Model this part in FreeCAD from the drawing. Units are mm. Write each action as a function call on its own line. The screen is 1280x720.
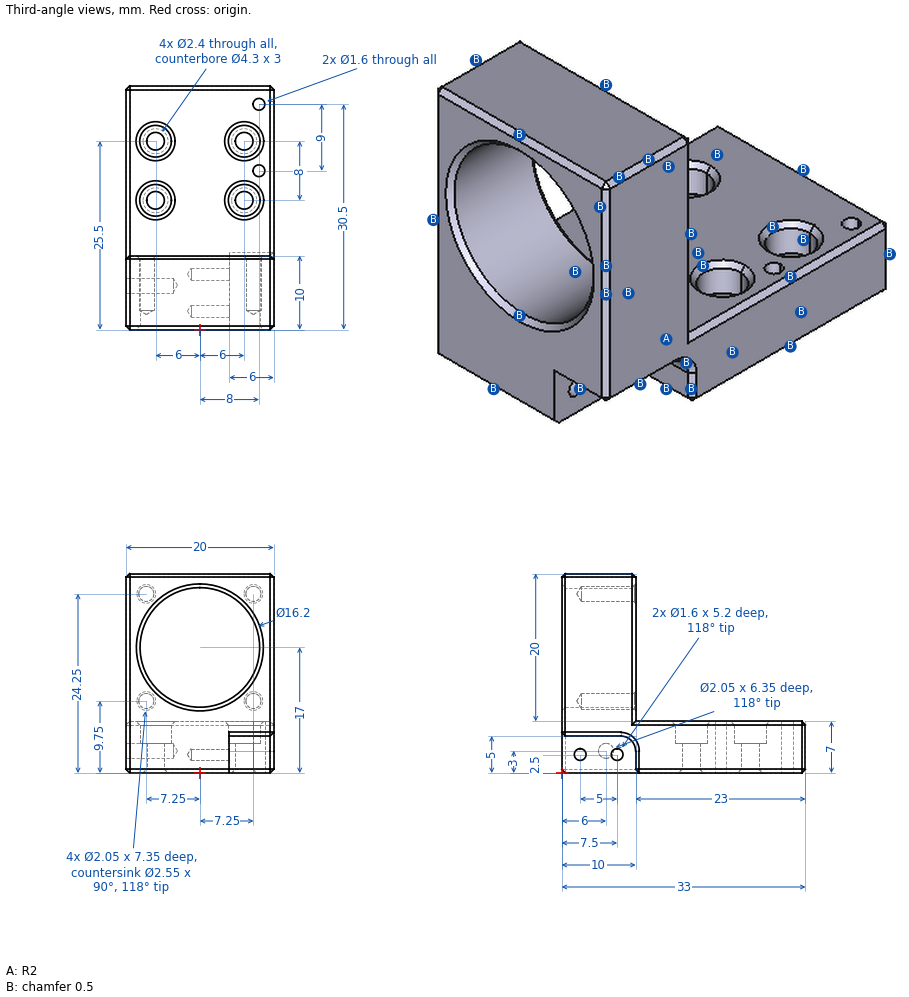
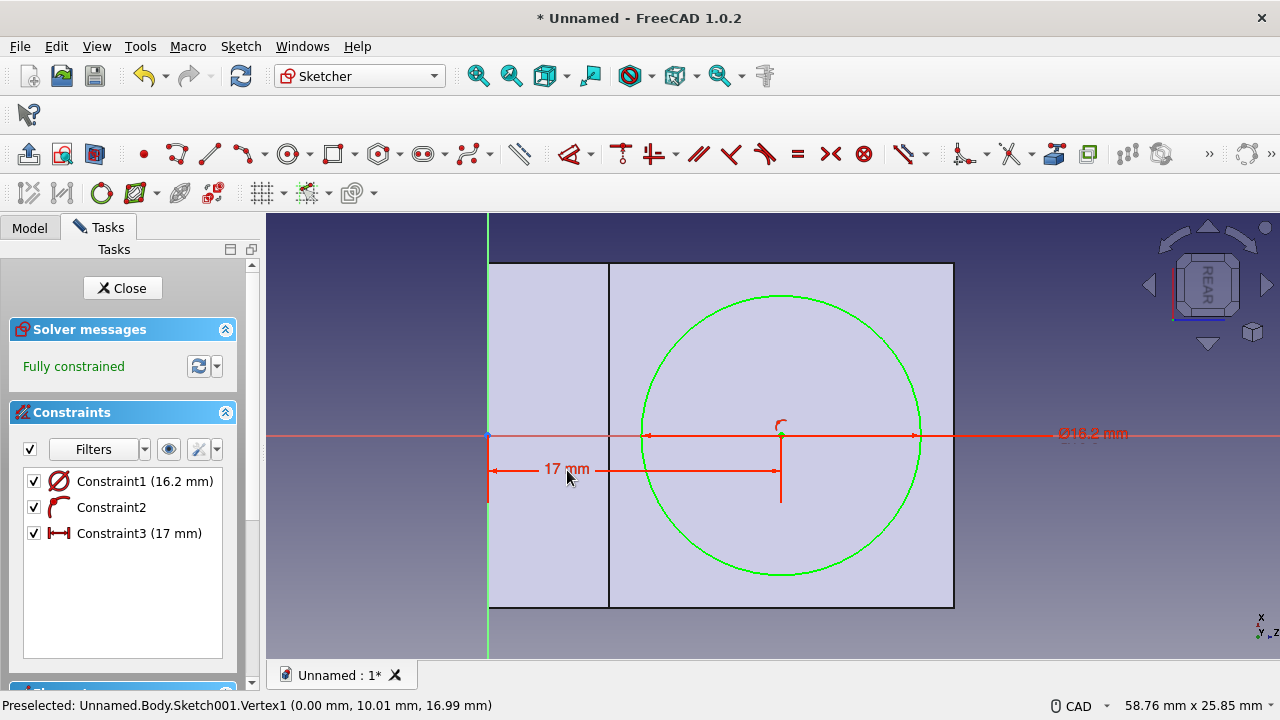
click(123, 288)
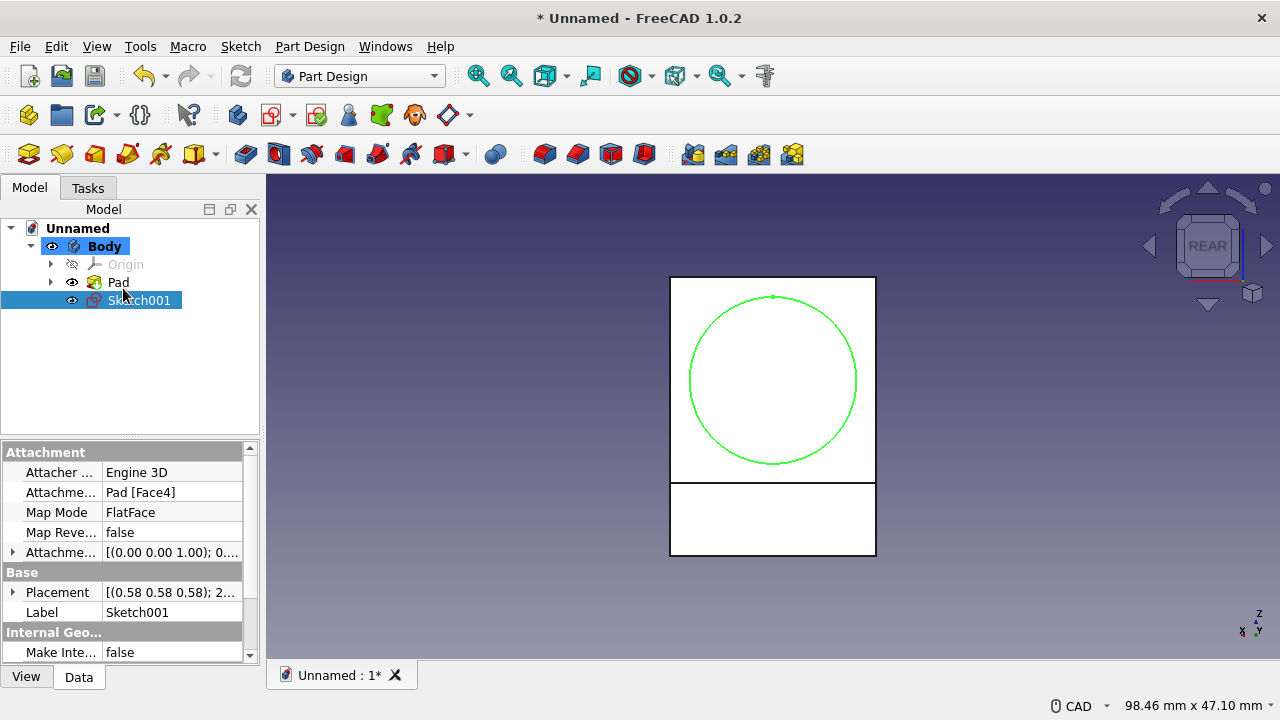
click(246, 154)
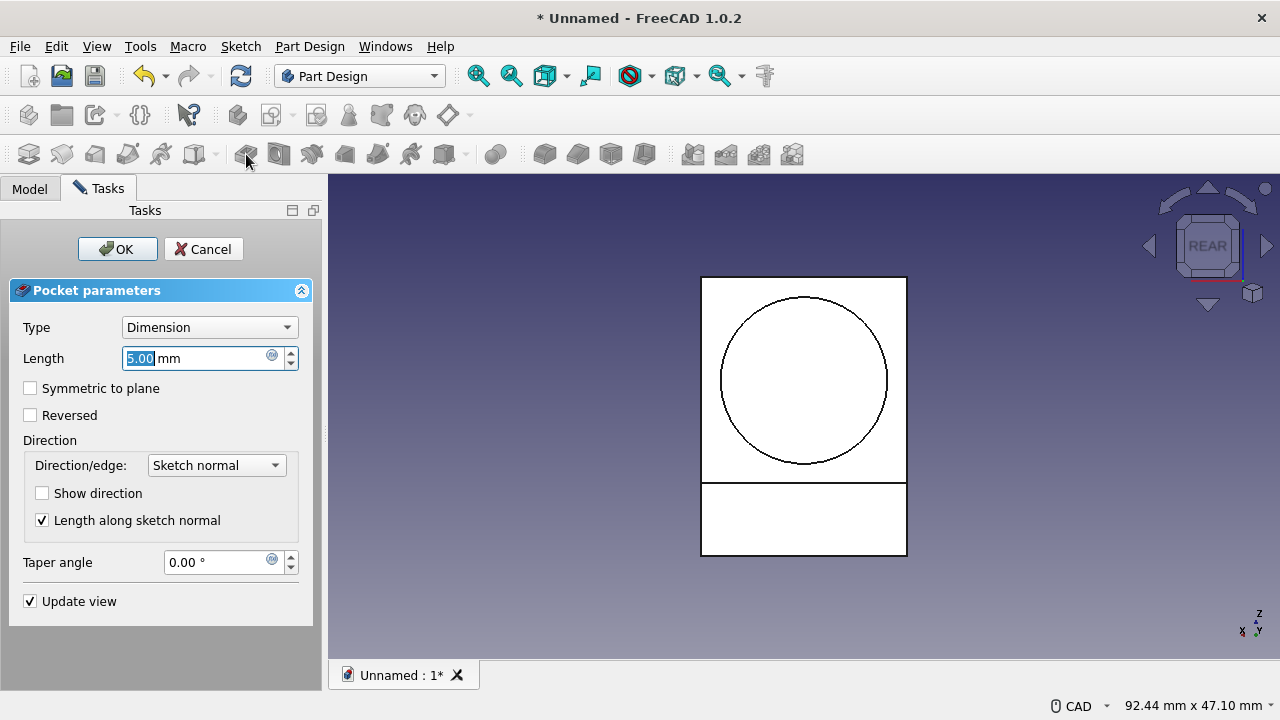
text(10)
key(Tab)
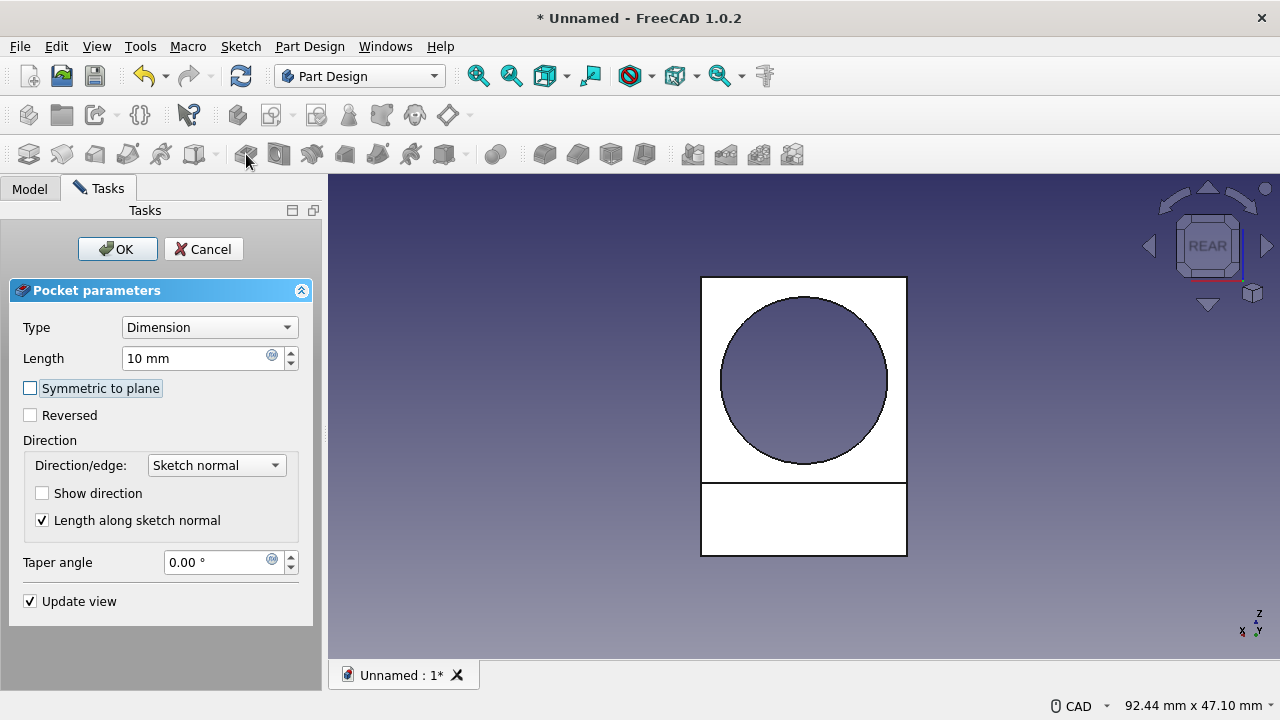
click(118, 249)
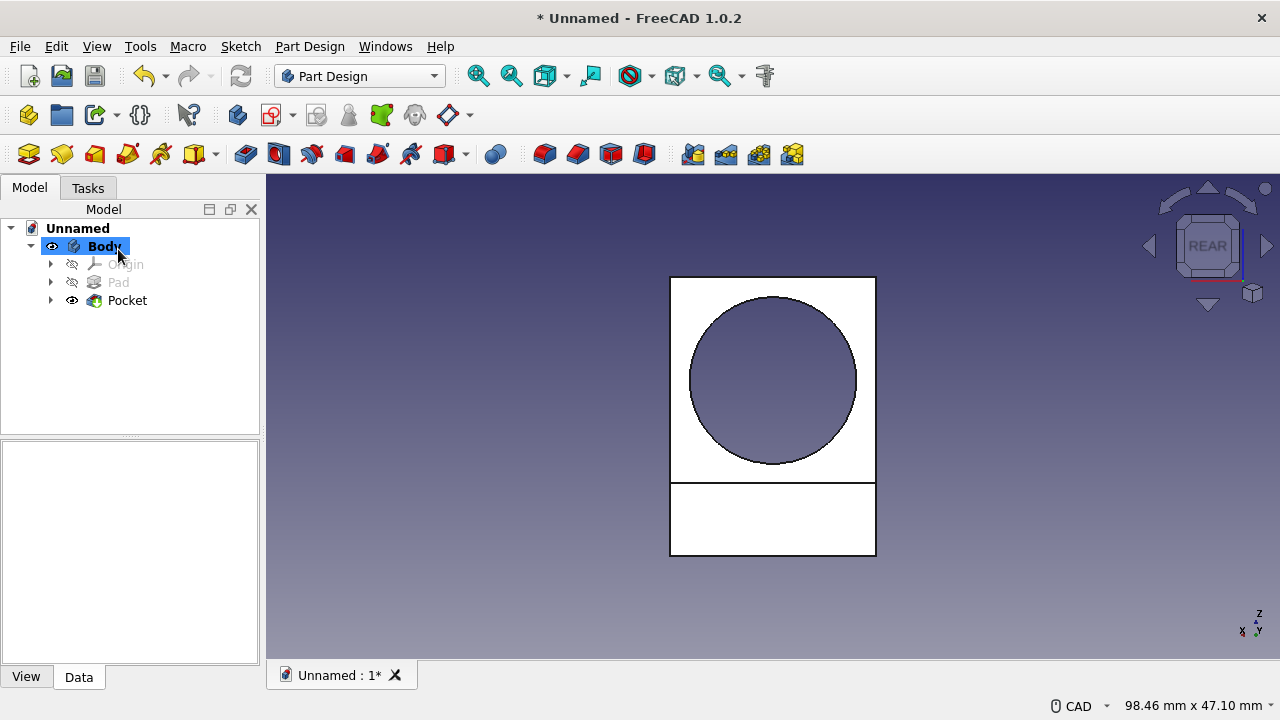
click(714, 468)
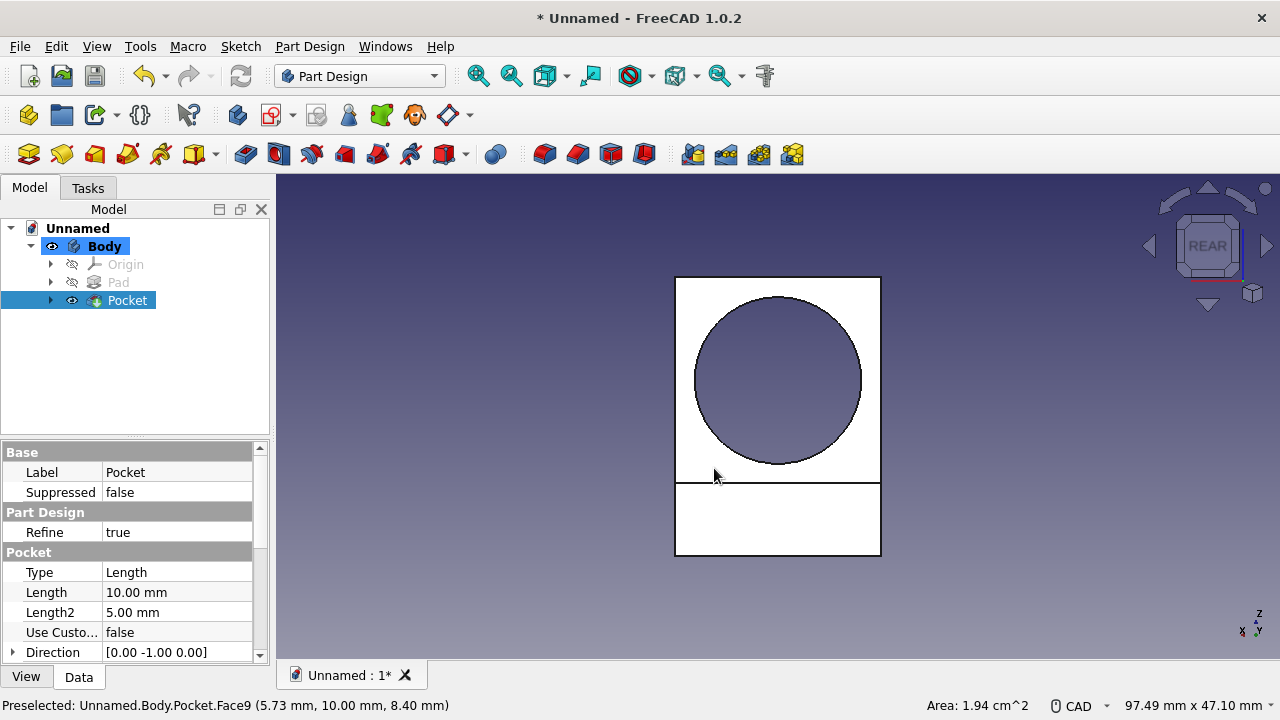
click(270, 116)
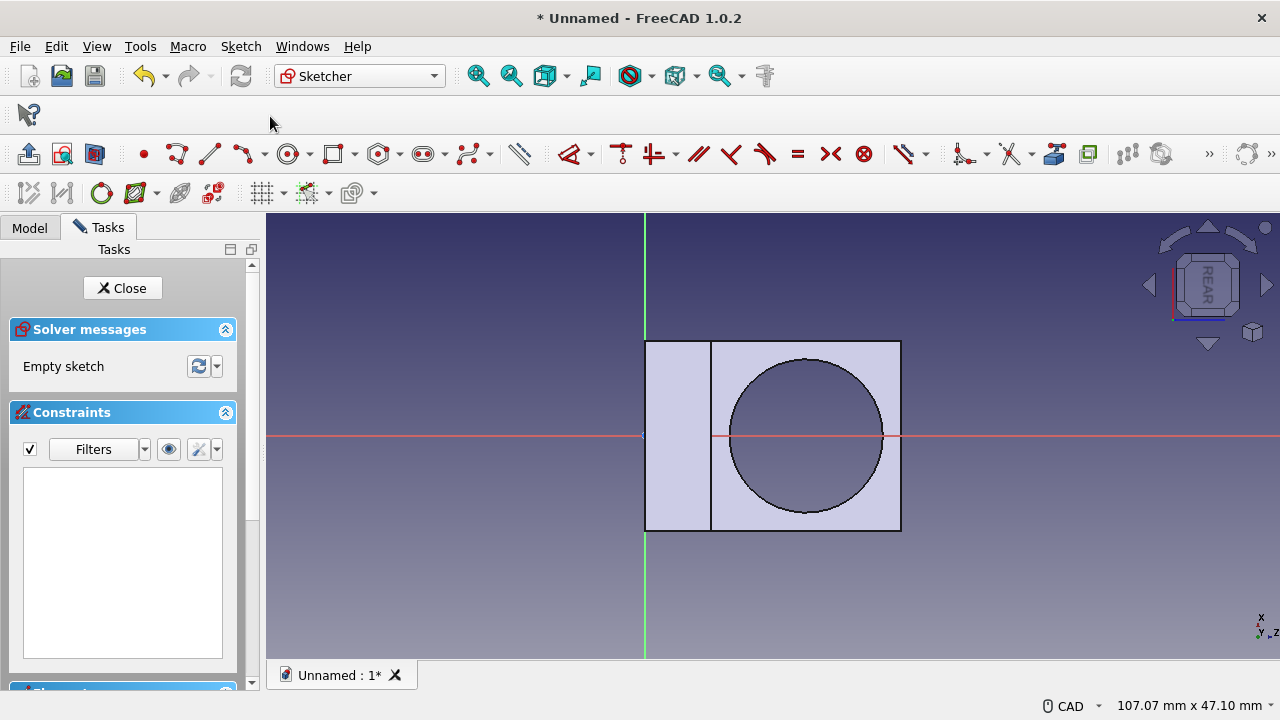
key(q)
key(s)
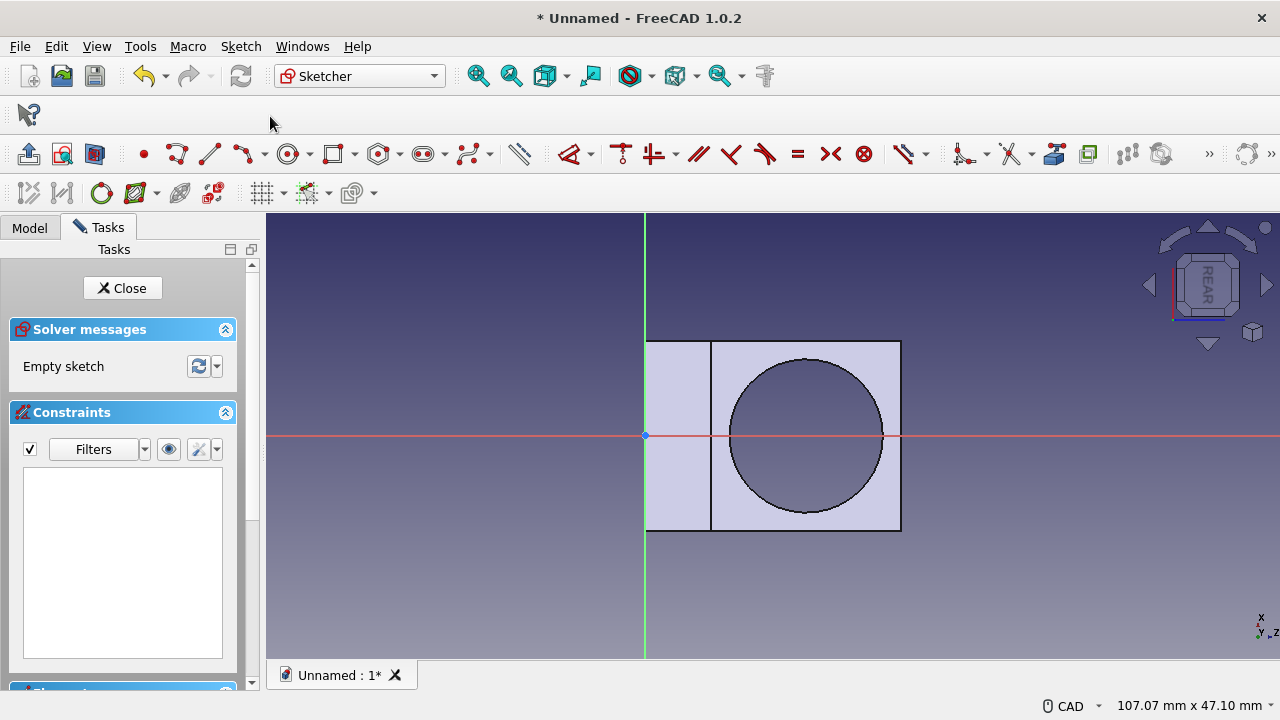
scroll(838, 436, up, 3)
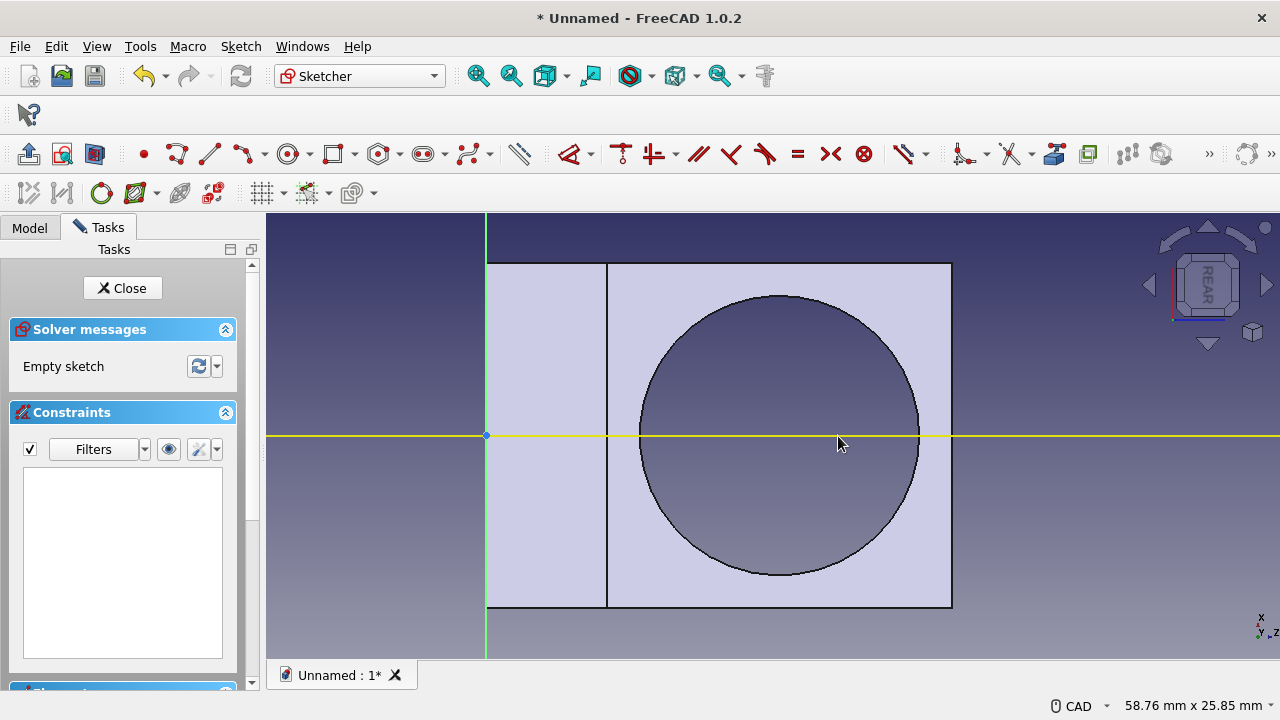
key(g)
key(c)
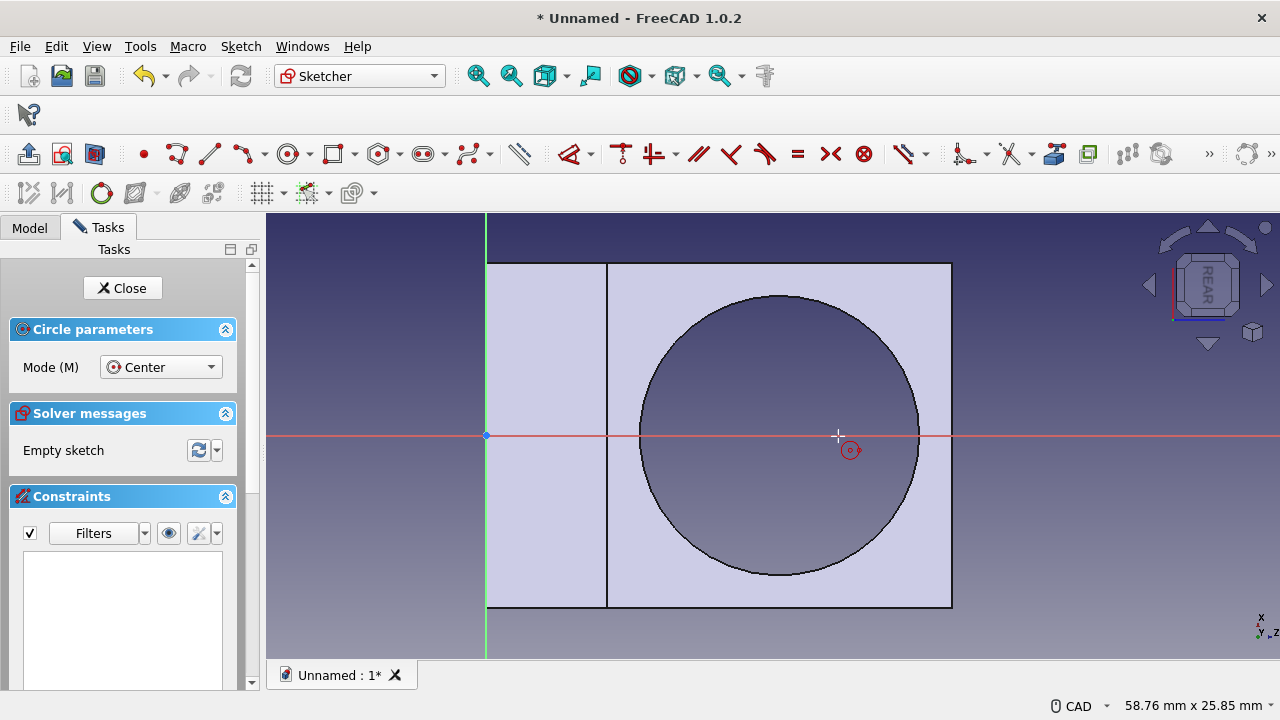
scroll(654, 561, up, 2)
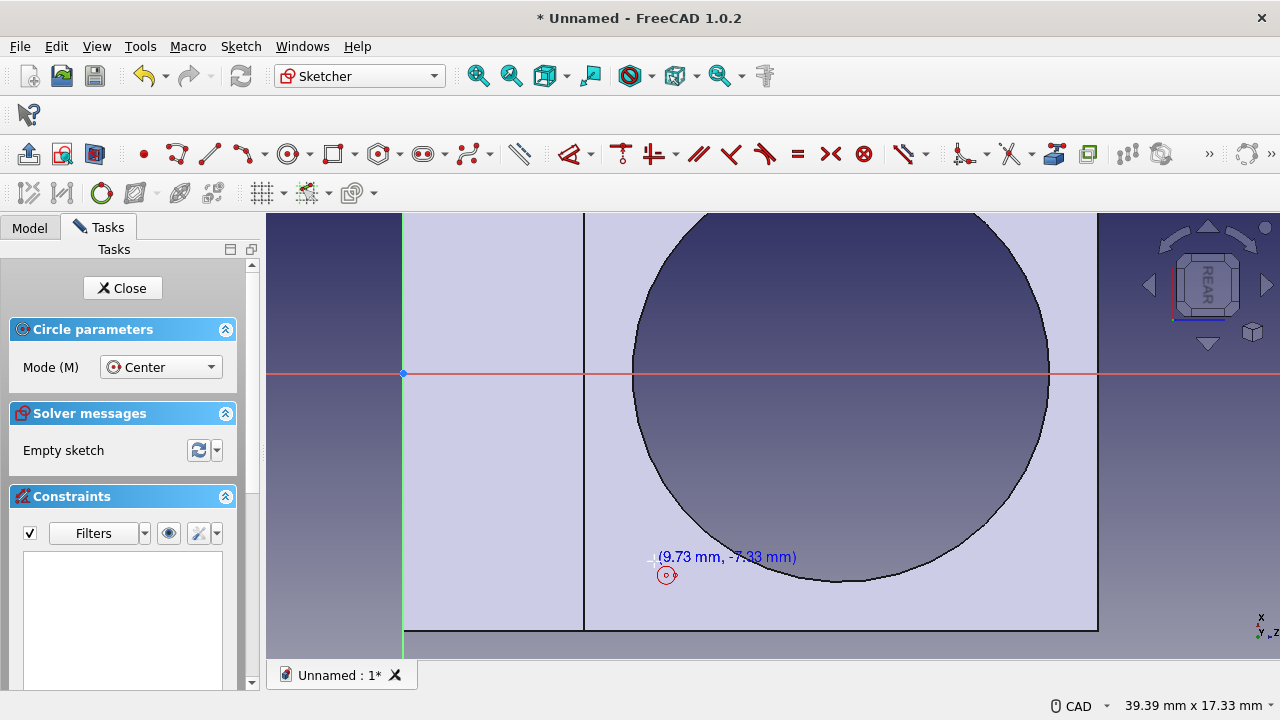
click(654, 560)
move(673, 541)